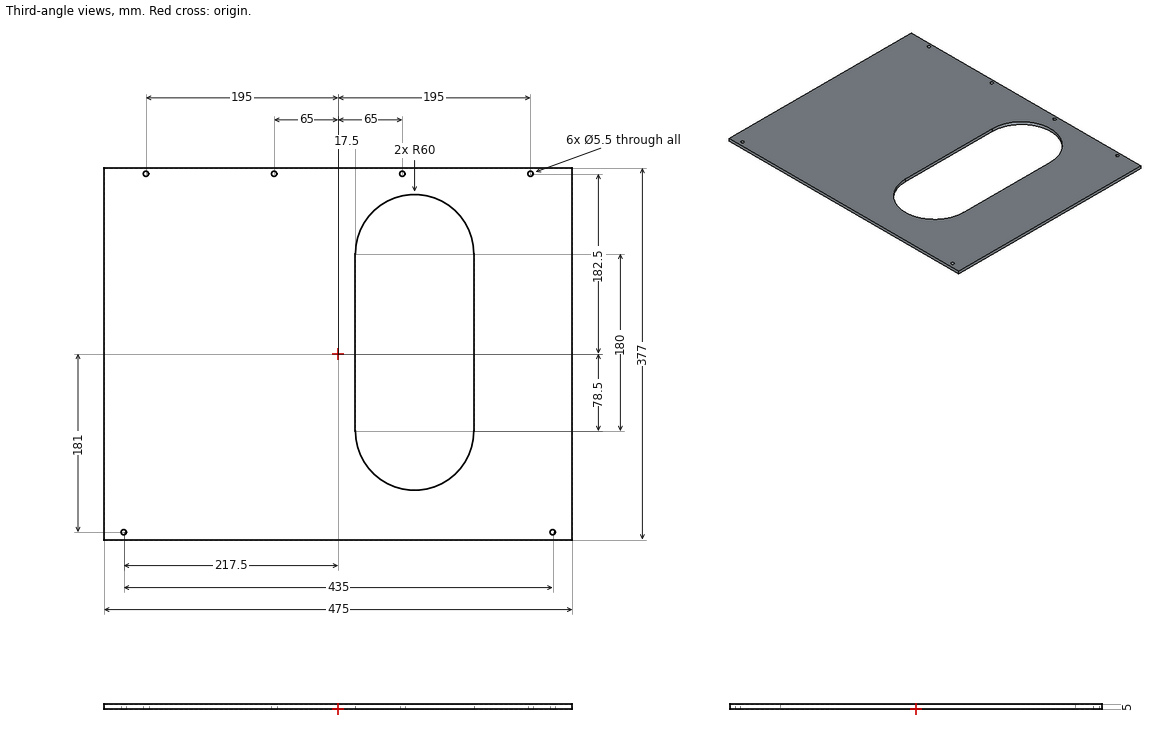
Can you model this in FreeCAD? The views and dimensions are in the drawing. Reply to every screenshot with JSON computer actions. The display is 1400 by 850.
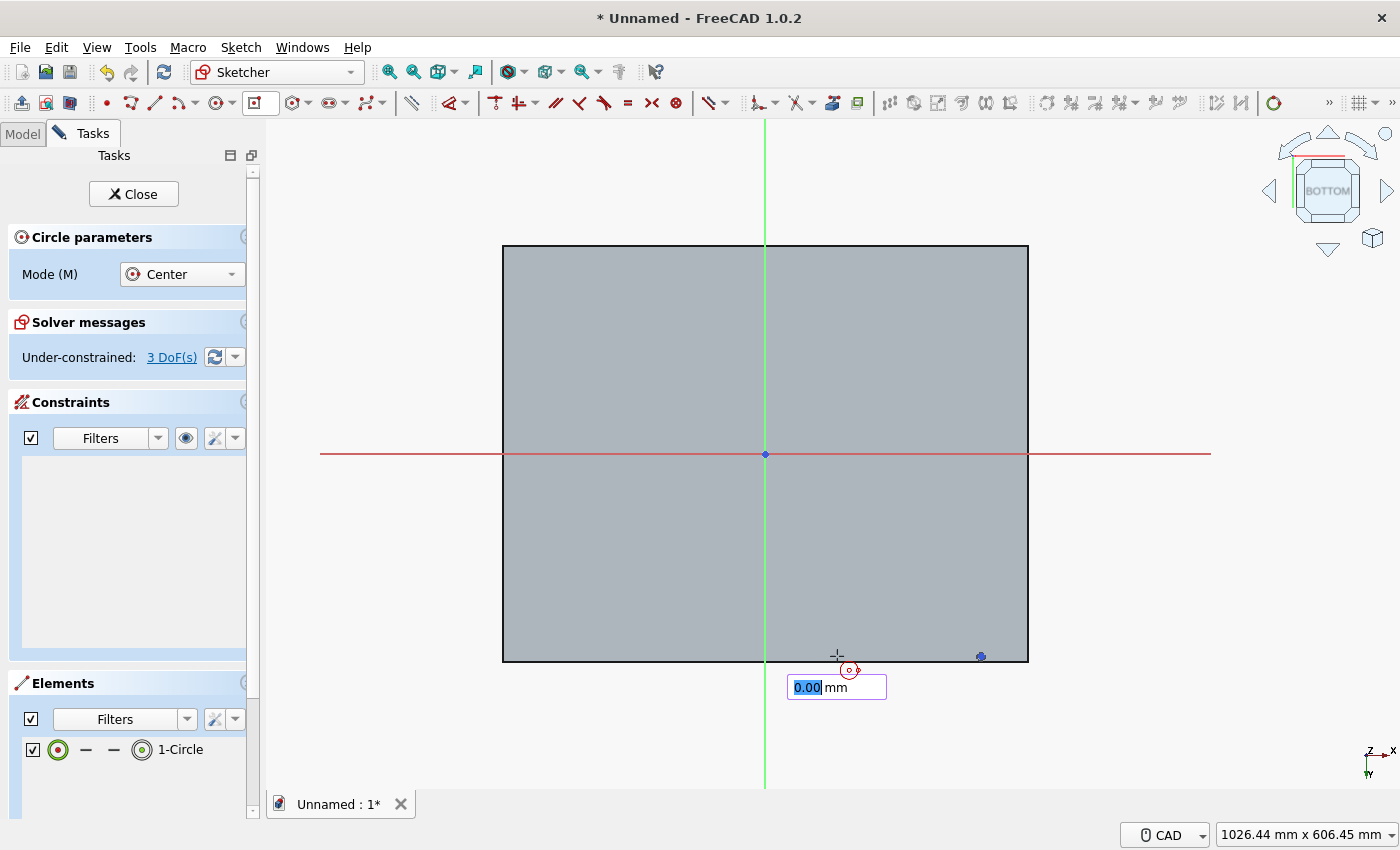
{"action": "scroll", "coordinate": [839, 653], "scroll_direction": "up", "scroll_amount": 9}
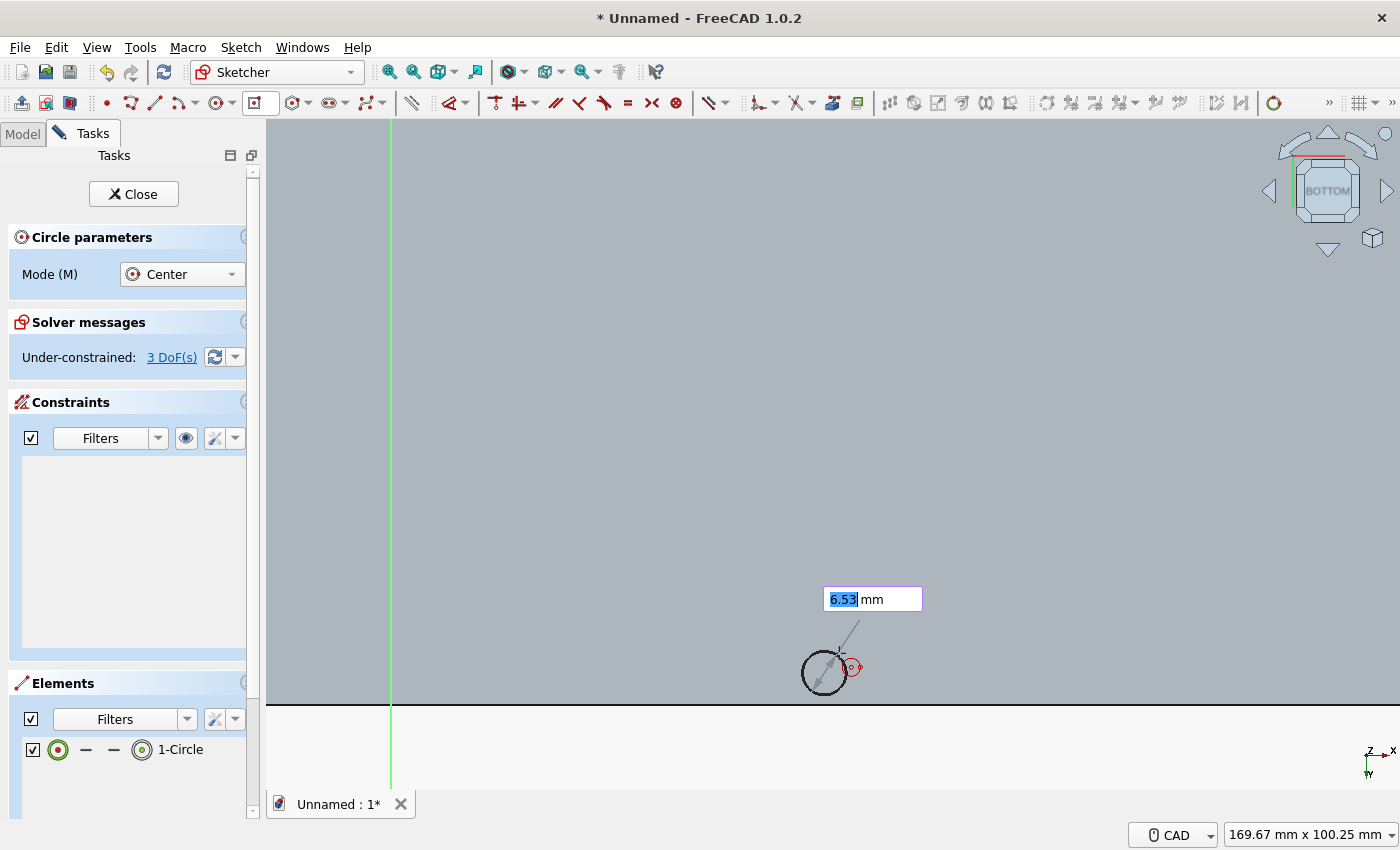
{"action": "left_click", "coordinate": [838, 652]}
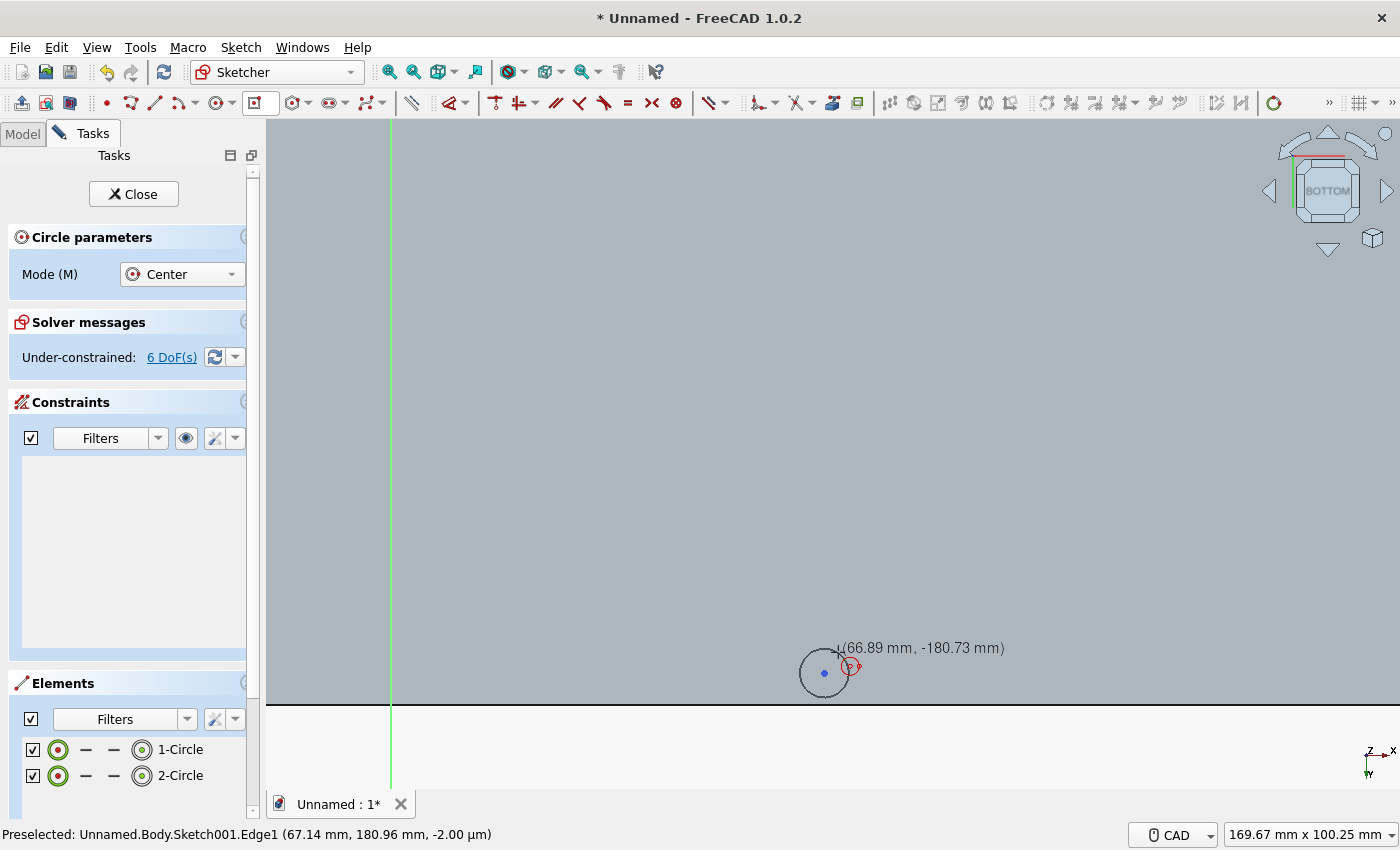
{"action": "scroll", "coordinate": [838, 653], "scroll_direction": "down", "scroll_amount": 9}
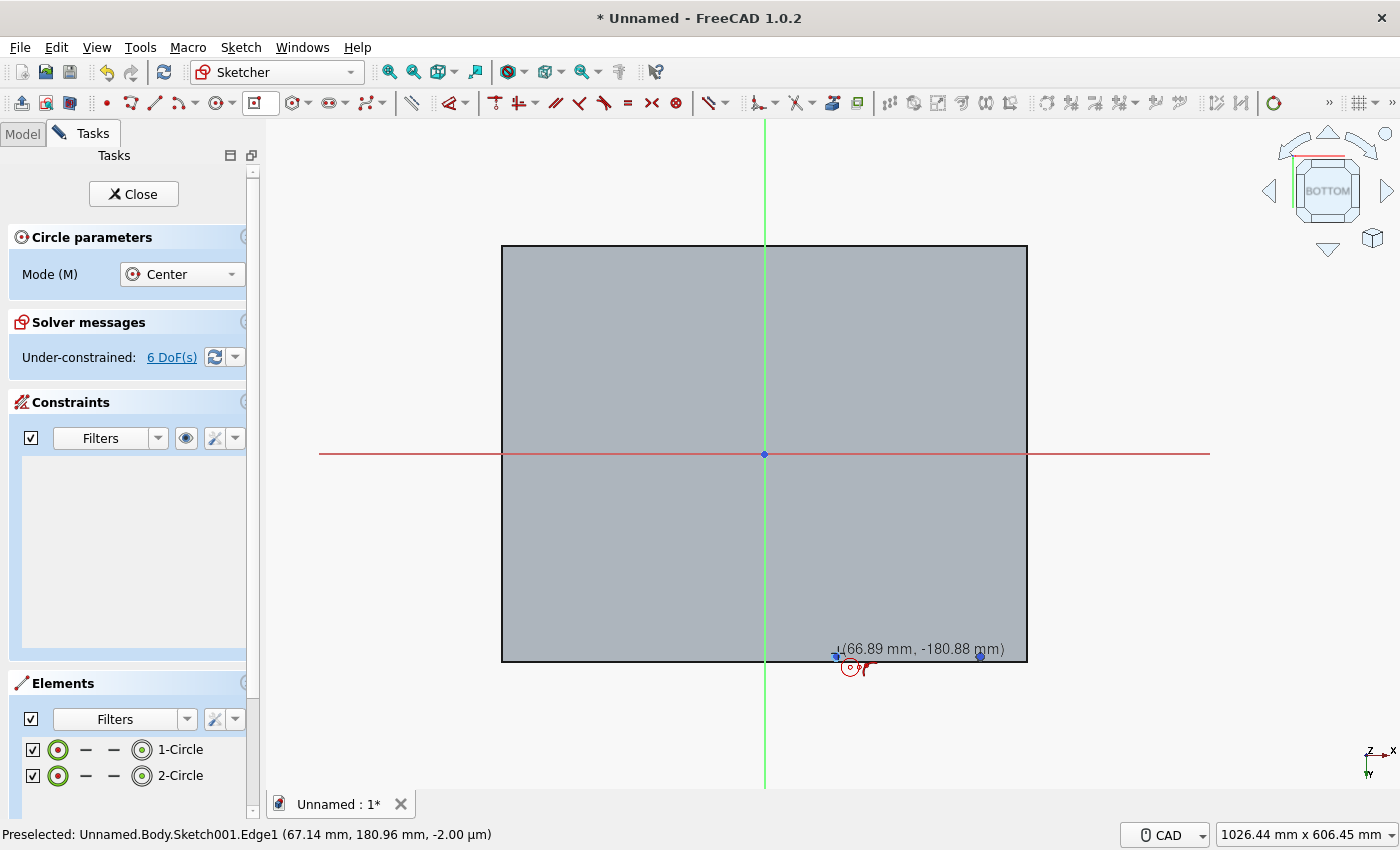
{"action": "scroll", "coordinate": [693, 656], "scroll_direction": "up", "scroll_amount": 11}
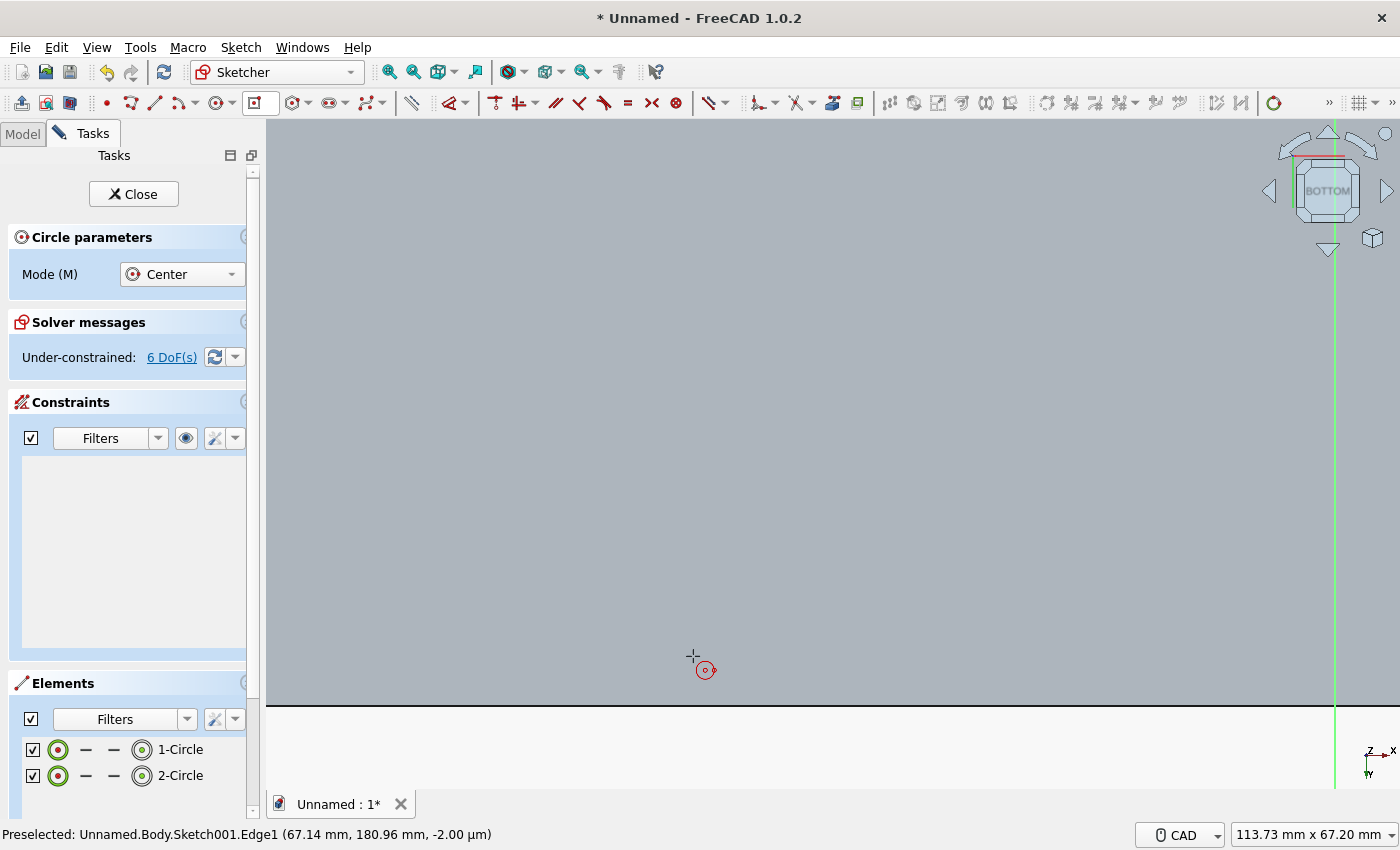
{"action": "scroll", "coordinate": [693, 656], "scroll_direction": "down", "scroll_amount": 11}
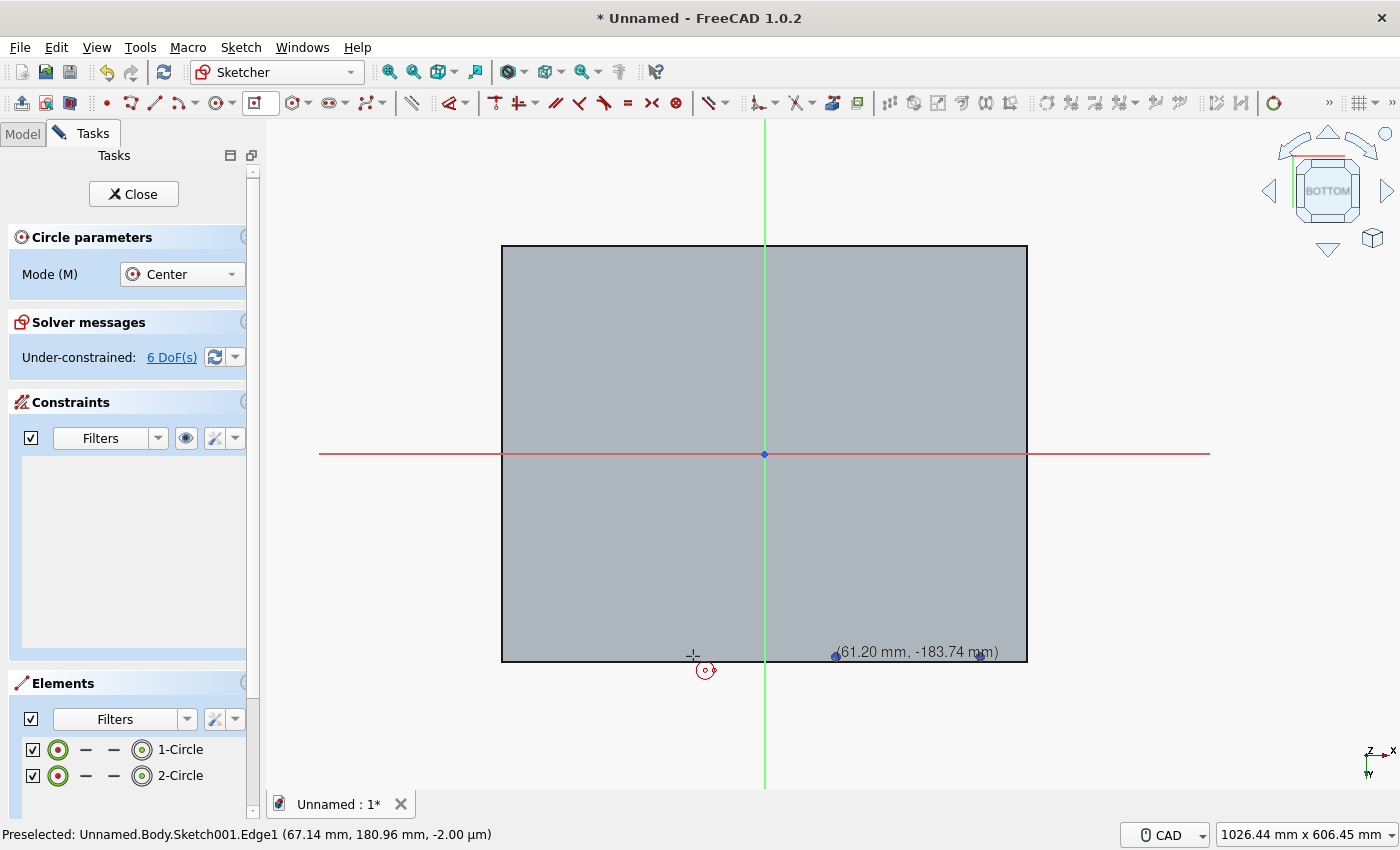
{"action": "left_click", "coordinate": [693, 656]}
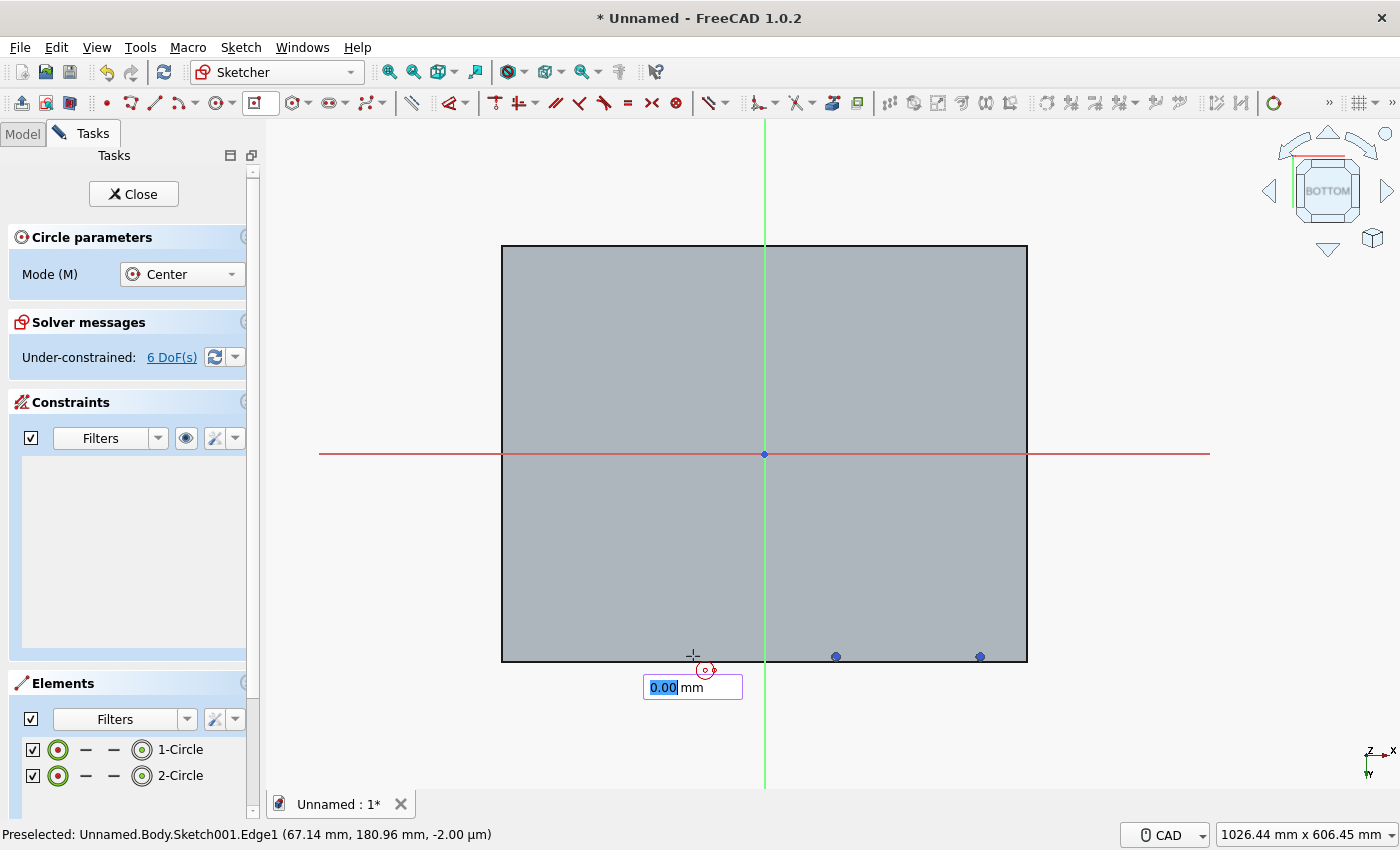
{"action": "scroll", "coordinate": [695, 653], "scroll_direction": "up", "scroll_amount": 9}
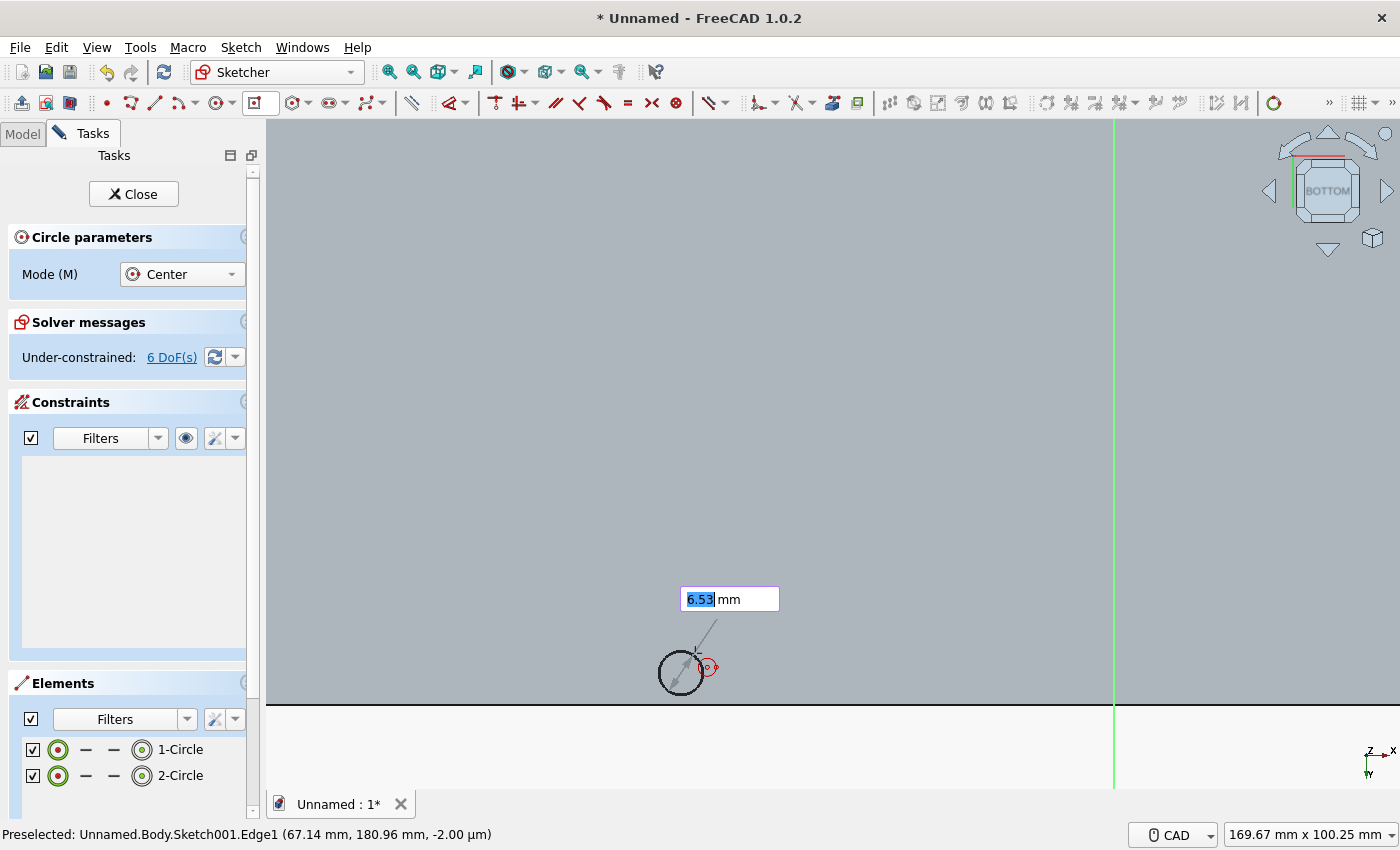
{"action": "left_click", "coordinate": [692, 652]}